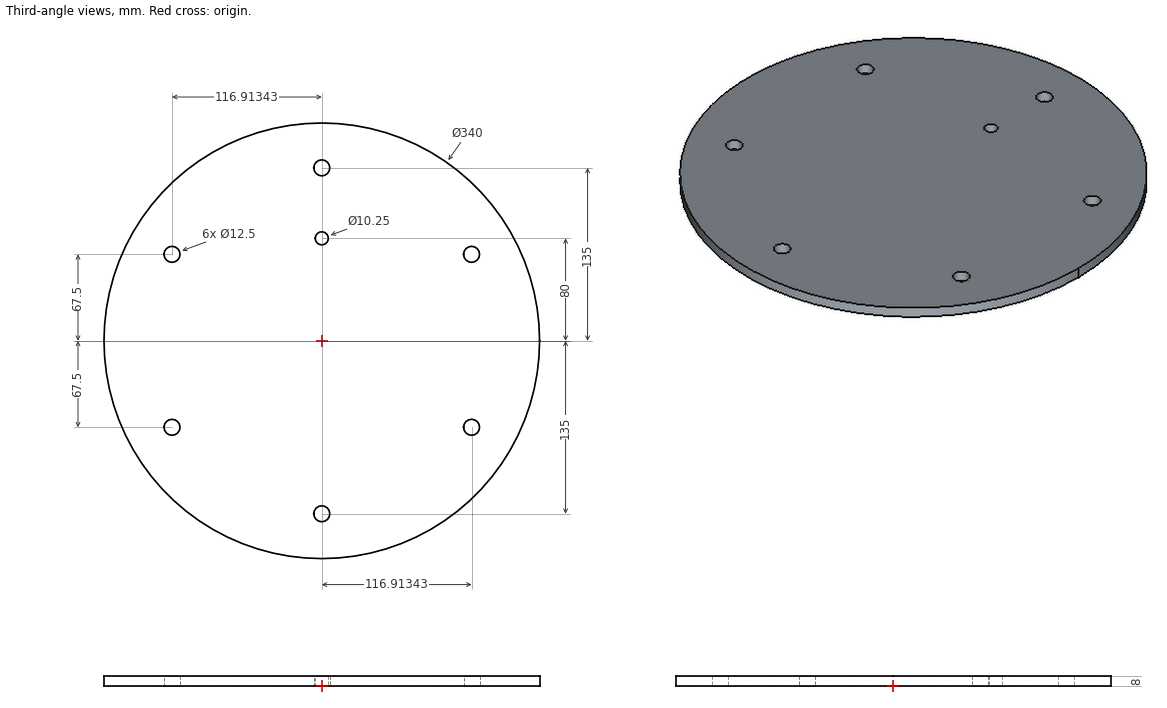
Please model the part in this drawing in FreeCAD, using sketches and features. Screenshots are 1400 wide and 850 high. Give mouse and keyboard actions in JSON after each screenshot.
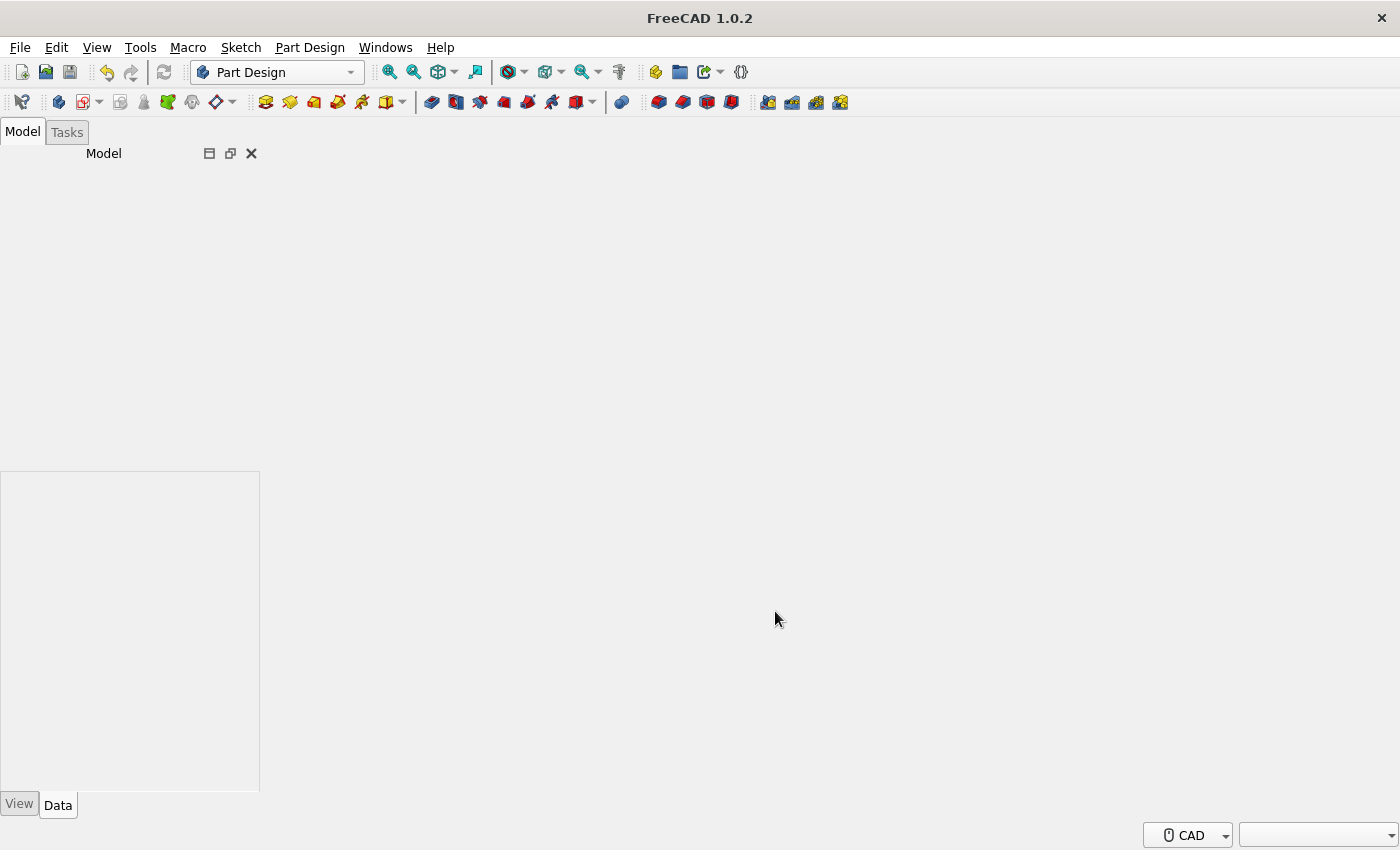
{"action": "left_click", "coordinate": [22, 72]}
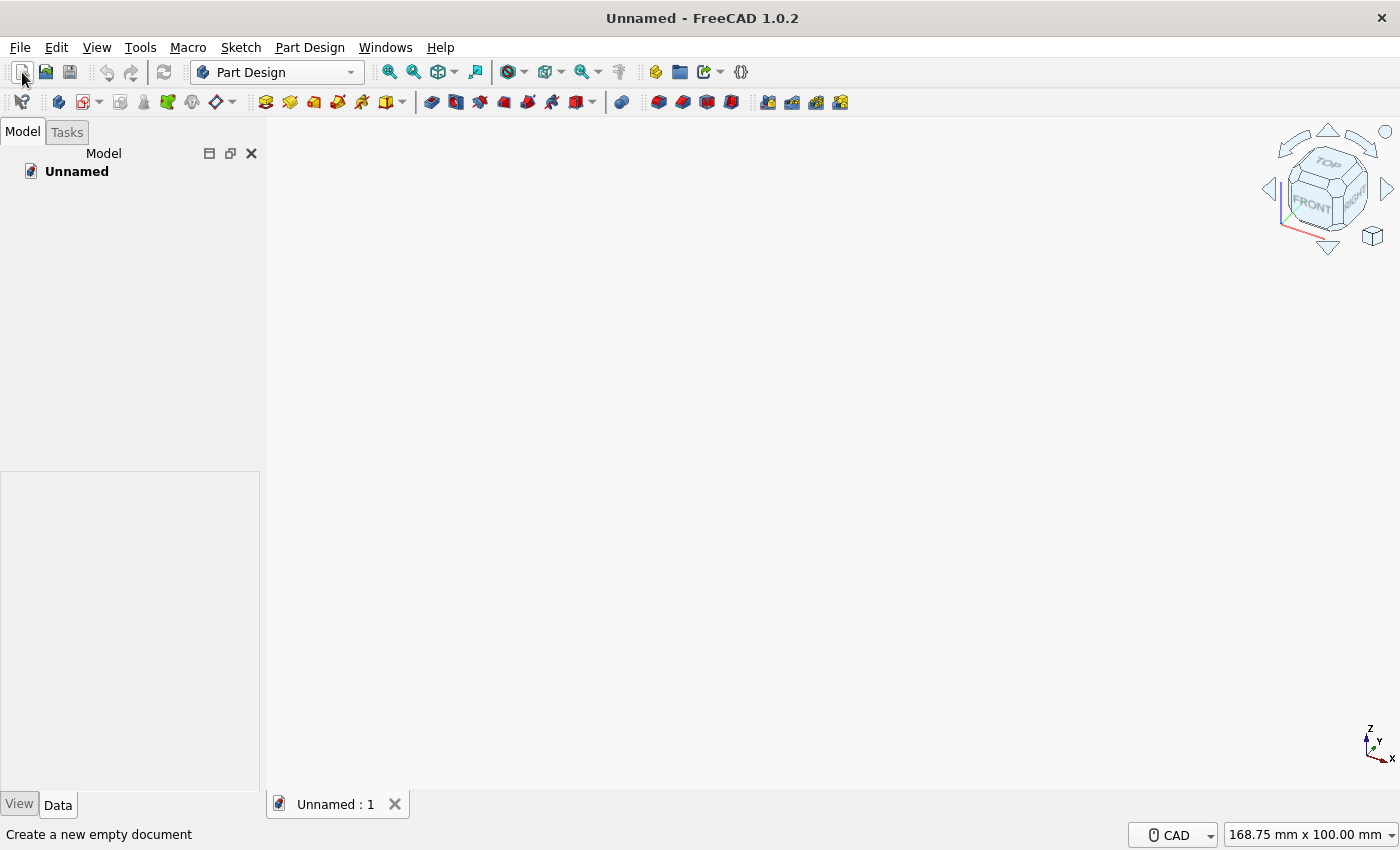
{"action": "left_click", "coordinate": [84, 102]}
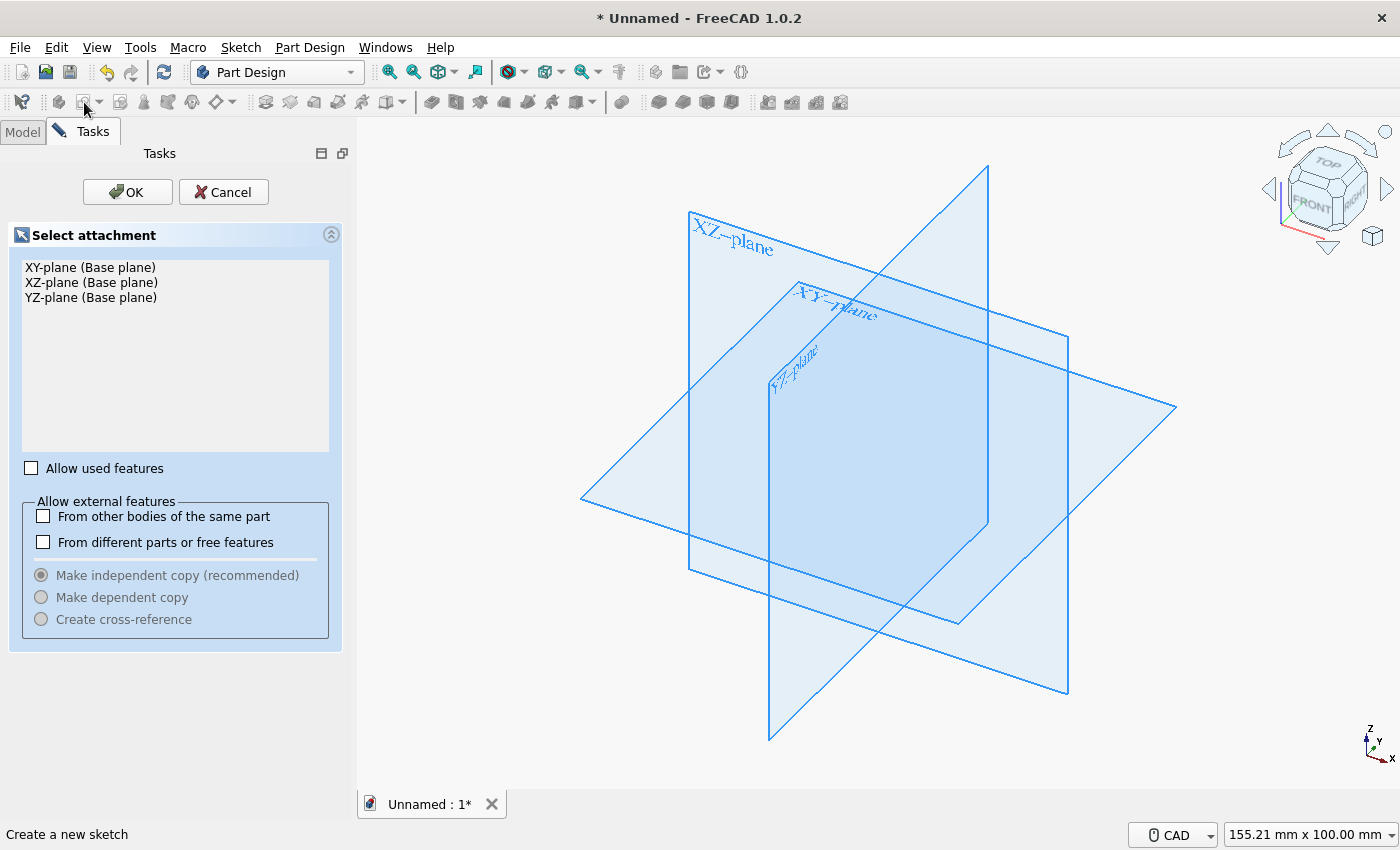
{"action": "left_click", "coordinate": [82, 268]}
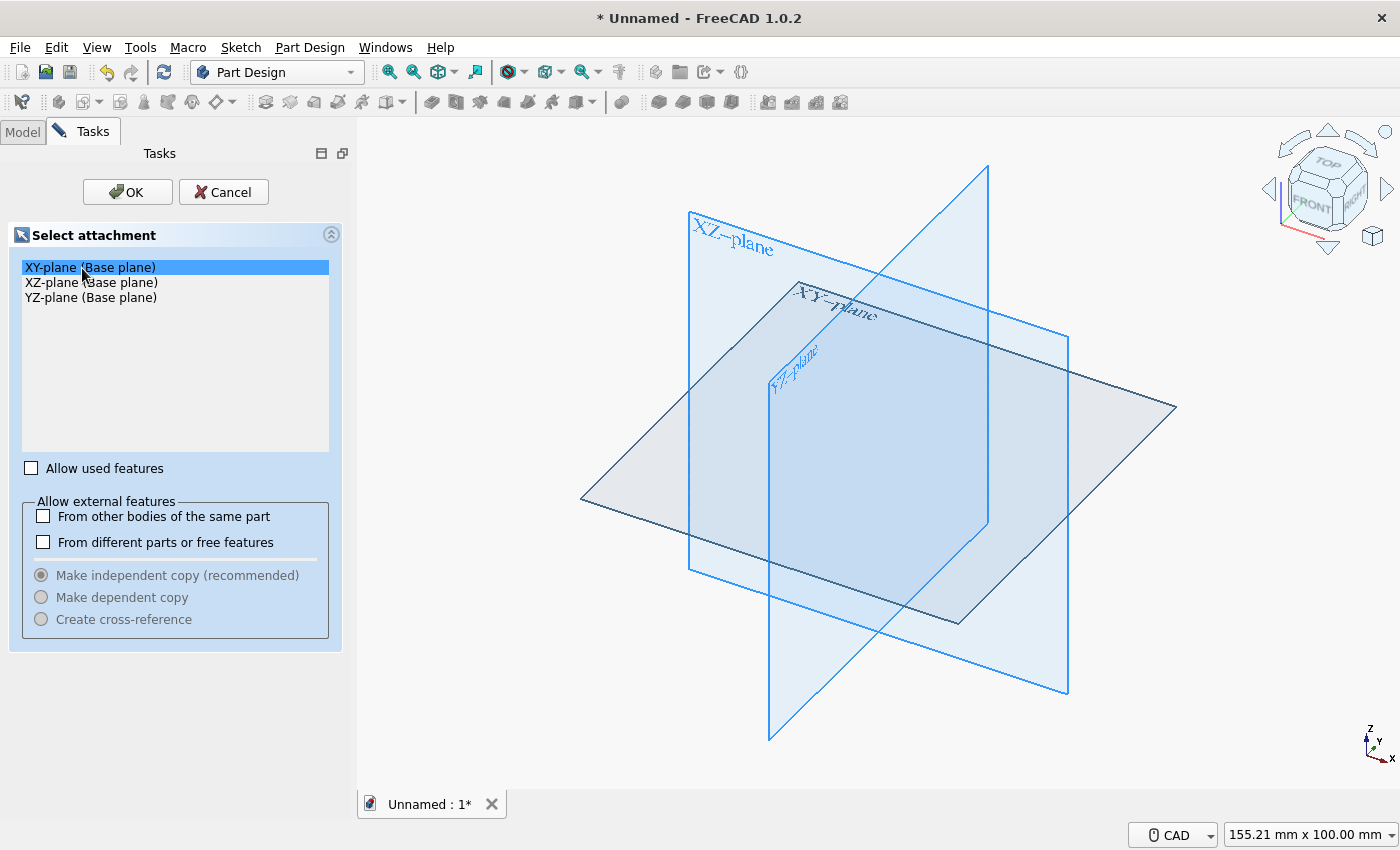
{"action": "left_click", "coordinate": [128, 192]}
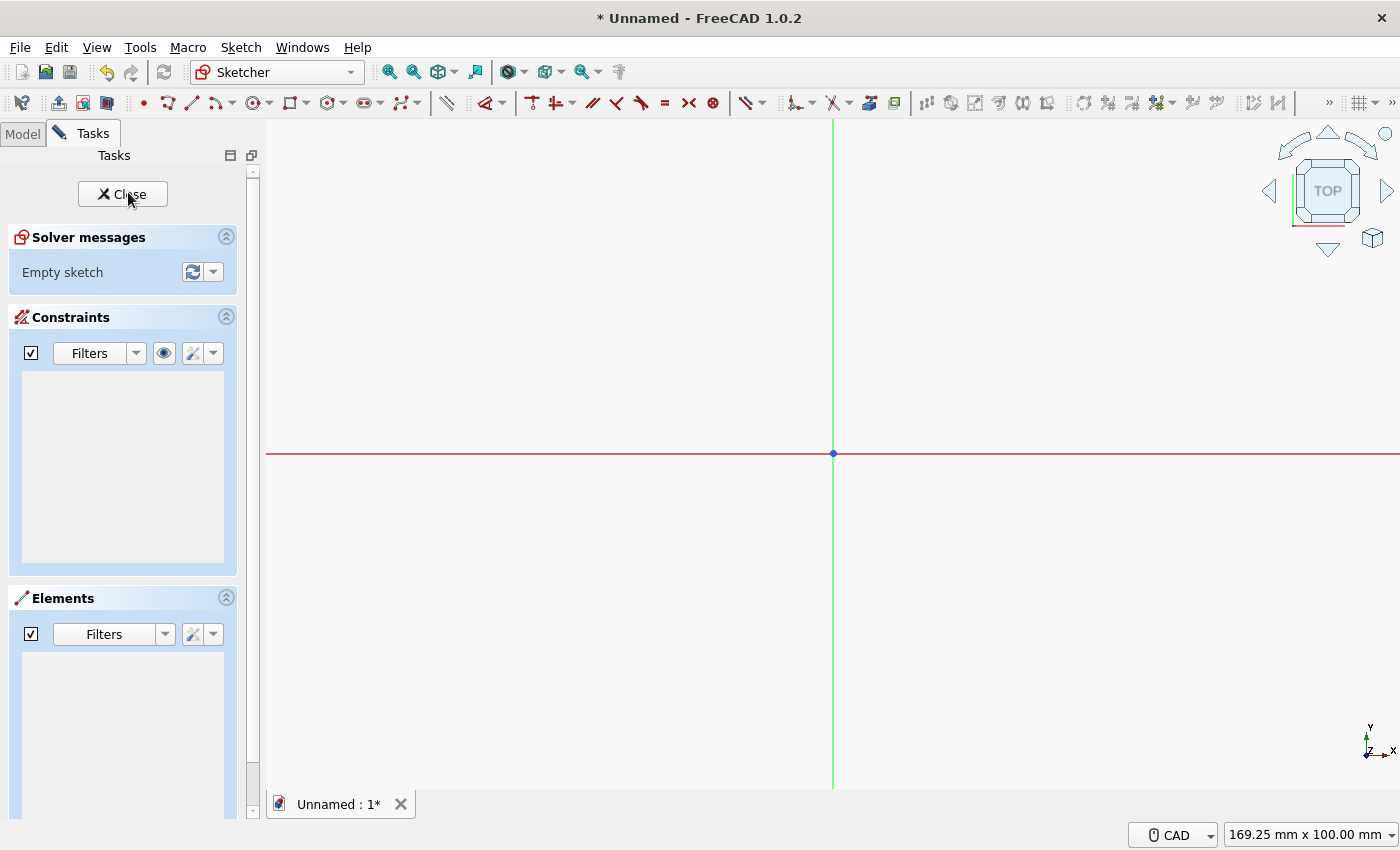
{"action": "scroll", "coordinate": [747, 454], "scroll_direction": "down", "scroll_amount": 8}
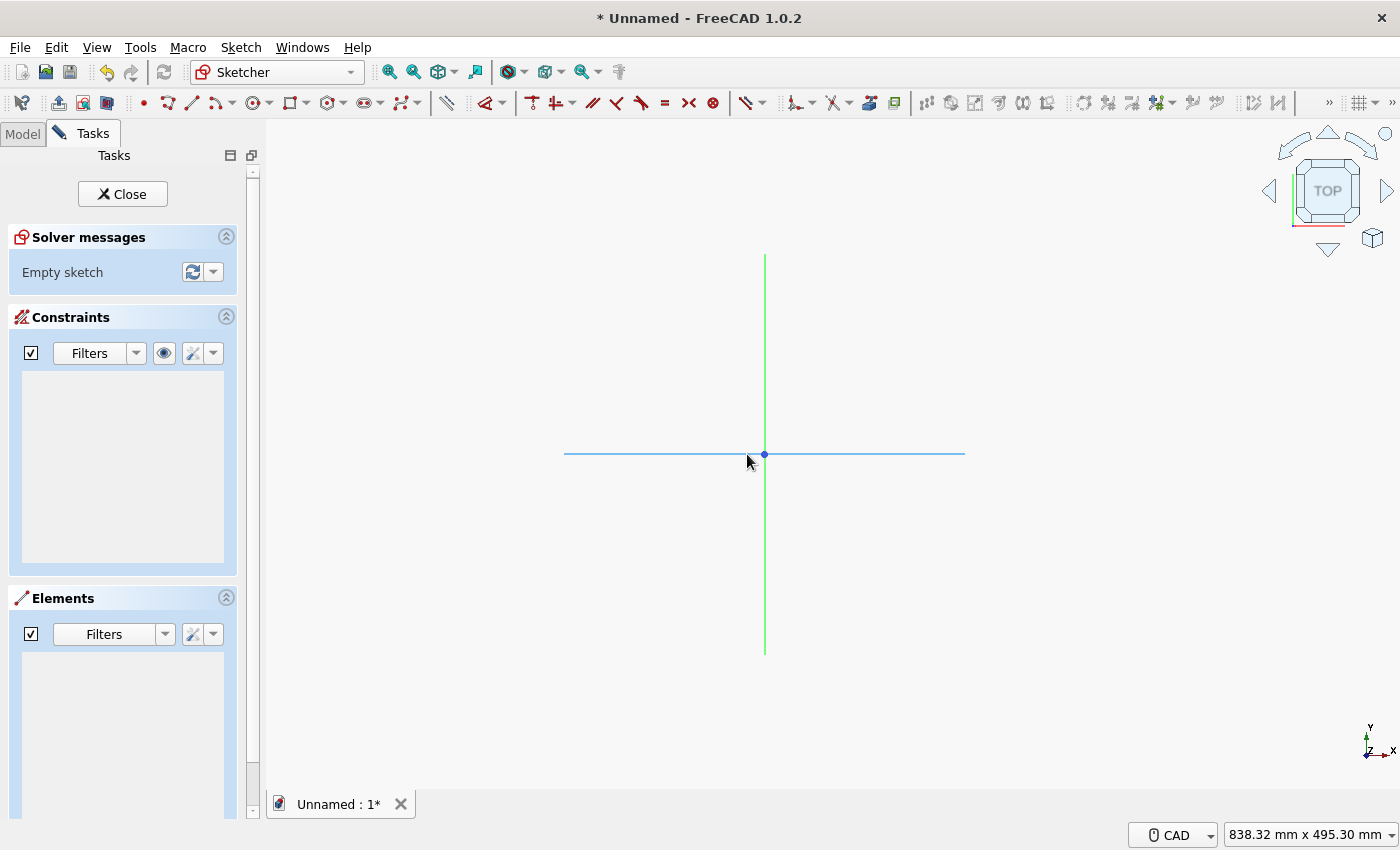
{"action": "left_click", "coordinate": [254, 104]}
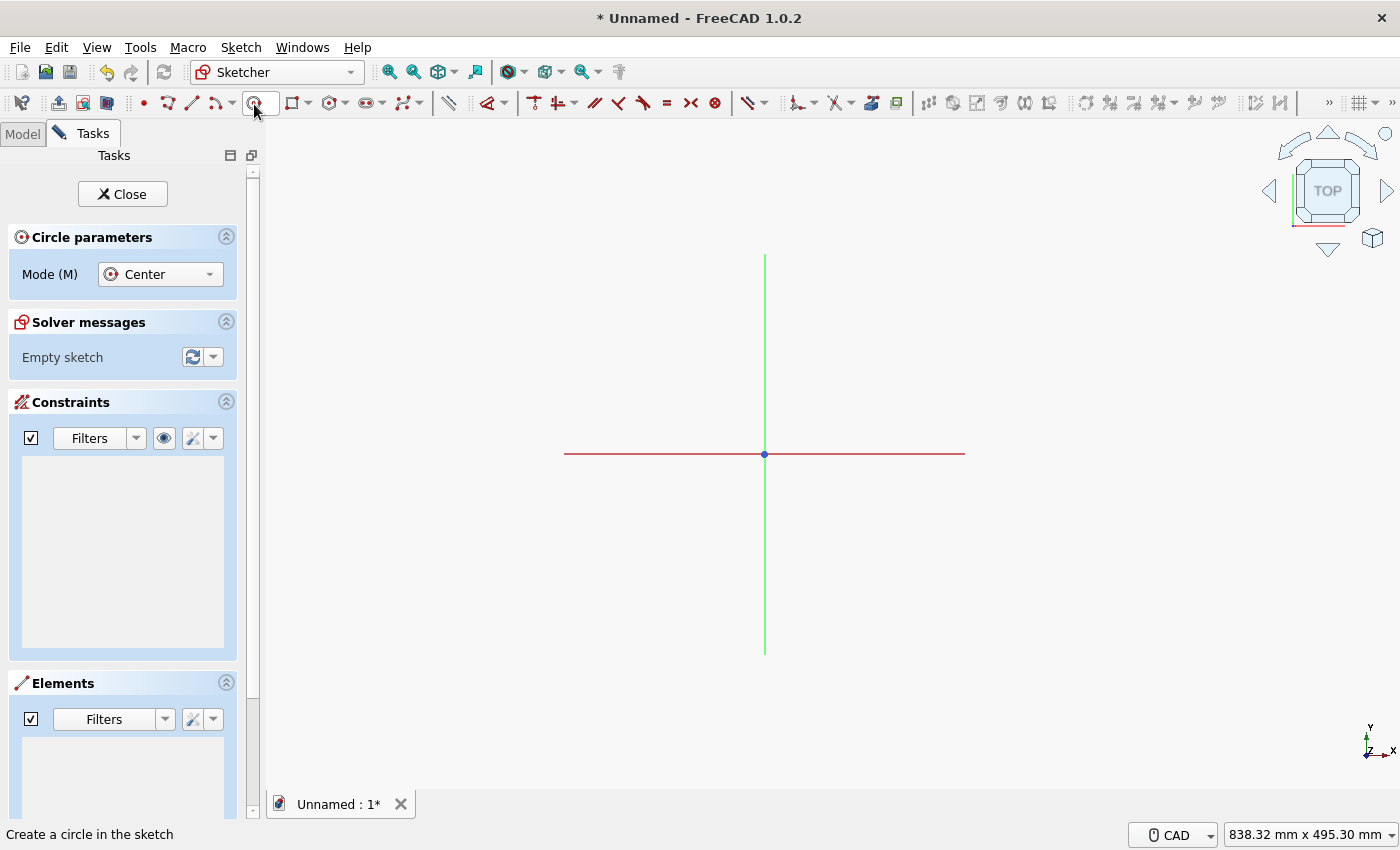
{"action": "left_click", "coordinate": [765, 454]}
{"action": "mouse_move", "coordinate": [927, 292]}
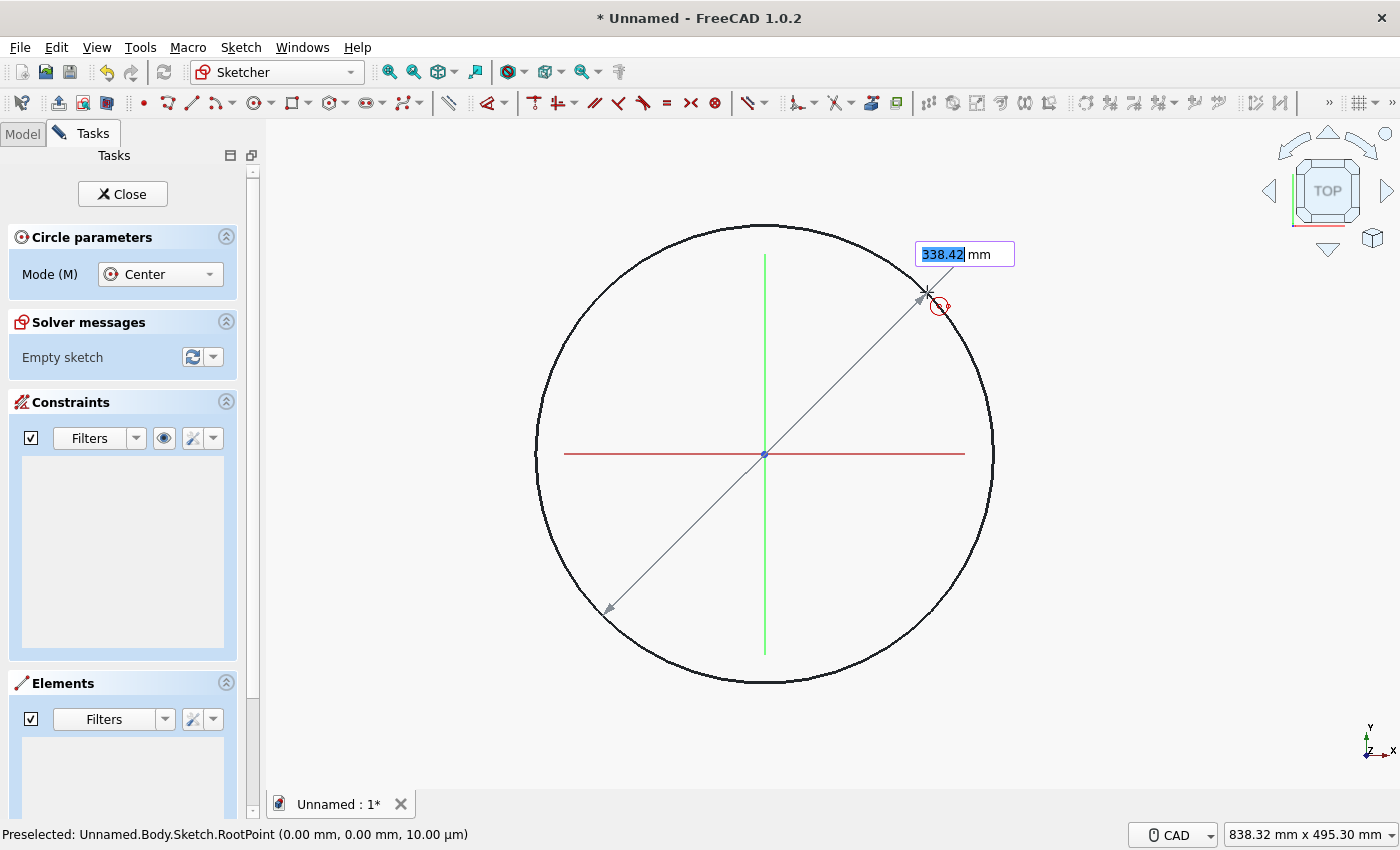
{"action": "type", "text": "340"}
{"action": "key", "text": "Return"}
{"action": "key", "text": "Escape"}